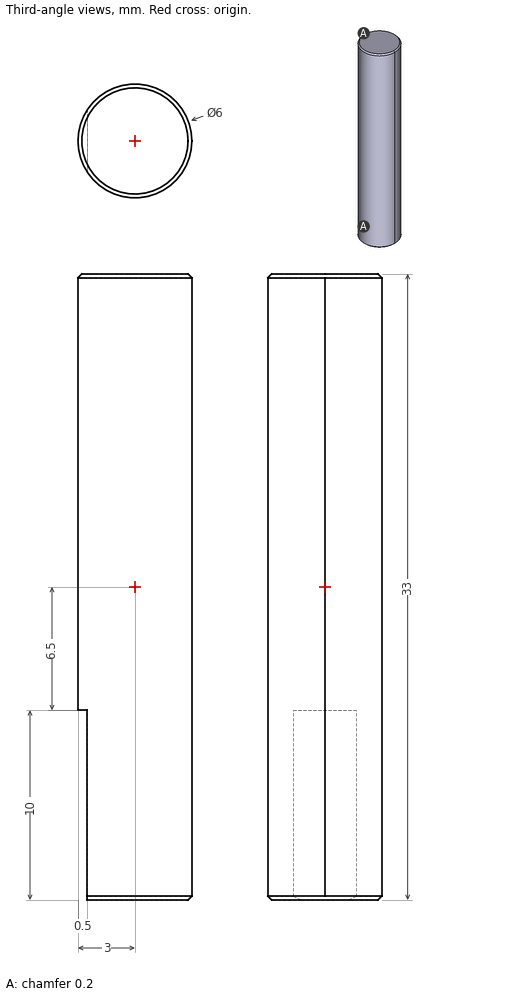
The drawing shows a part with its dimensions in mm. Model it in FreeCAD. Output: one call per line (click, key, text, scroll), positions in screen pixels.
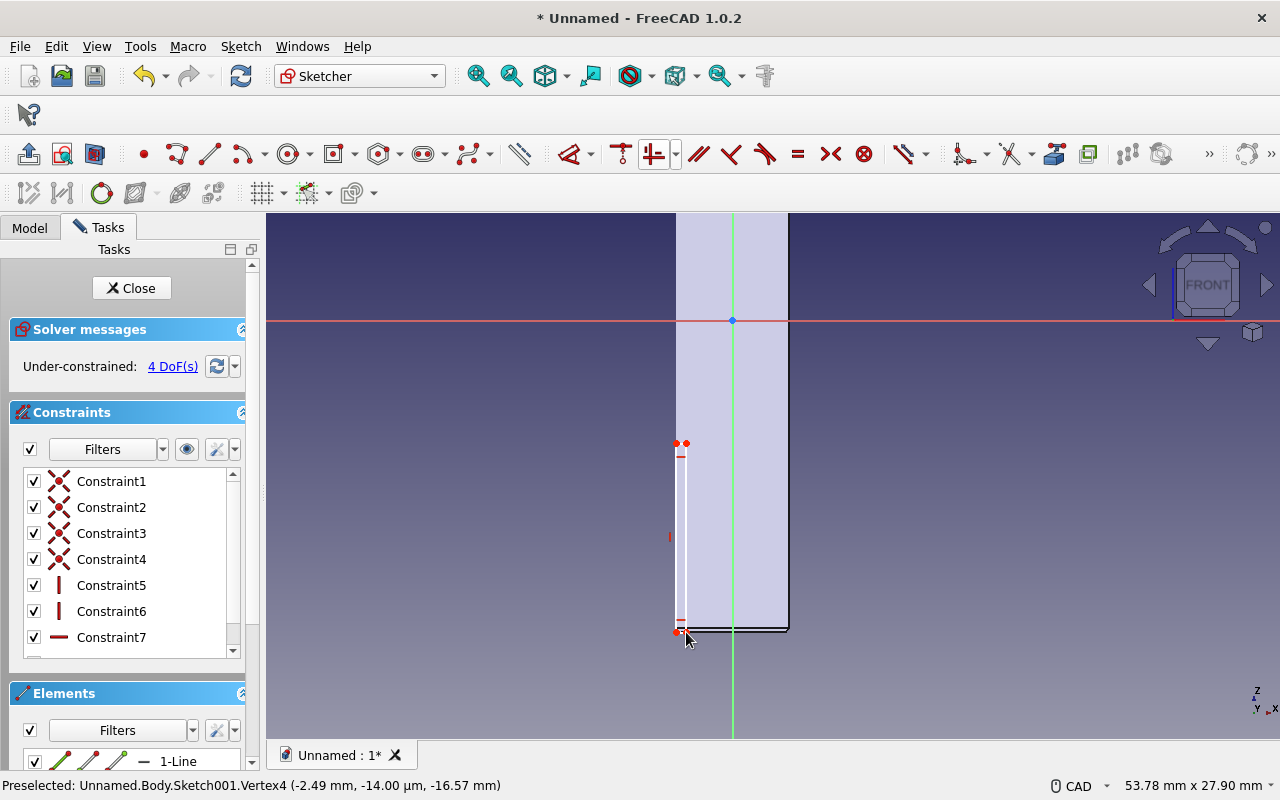
click(568, 154)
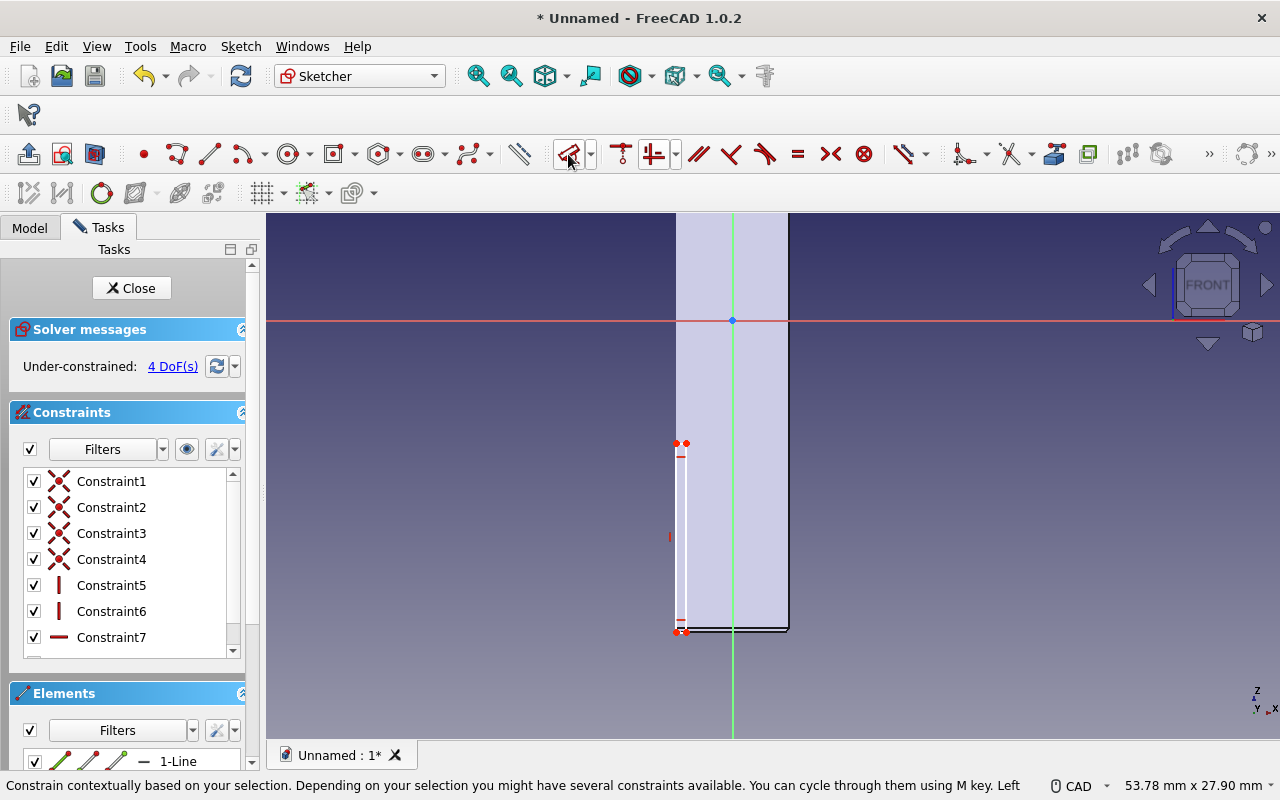
scroll(676, 500, up, 2)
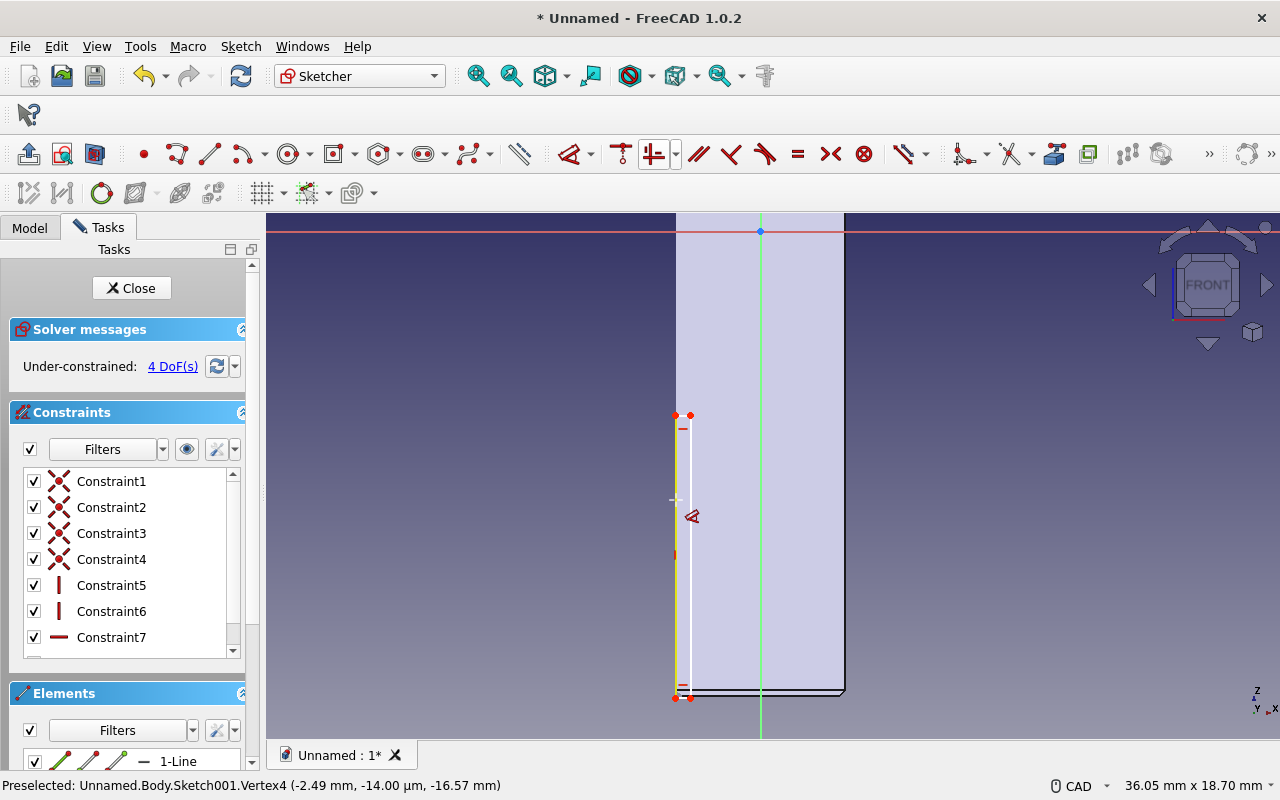
click(676, 500)
click(642, 557)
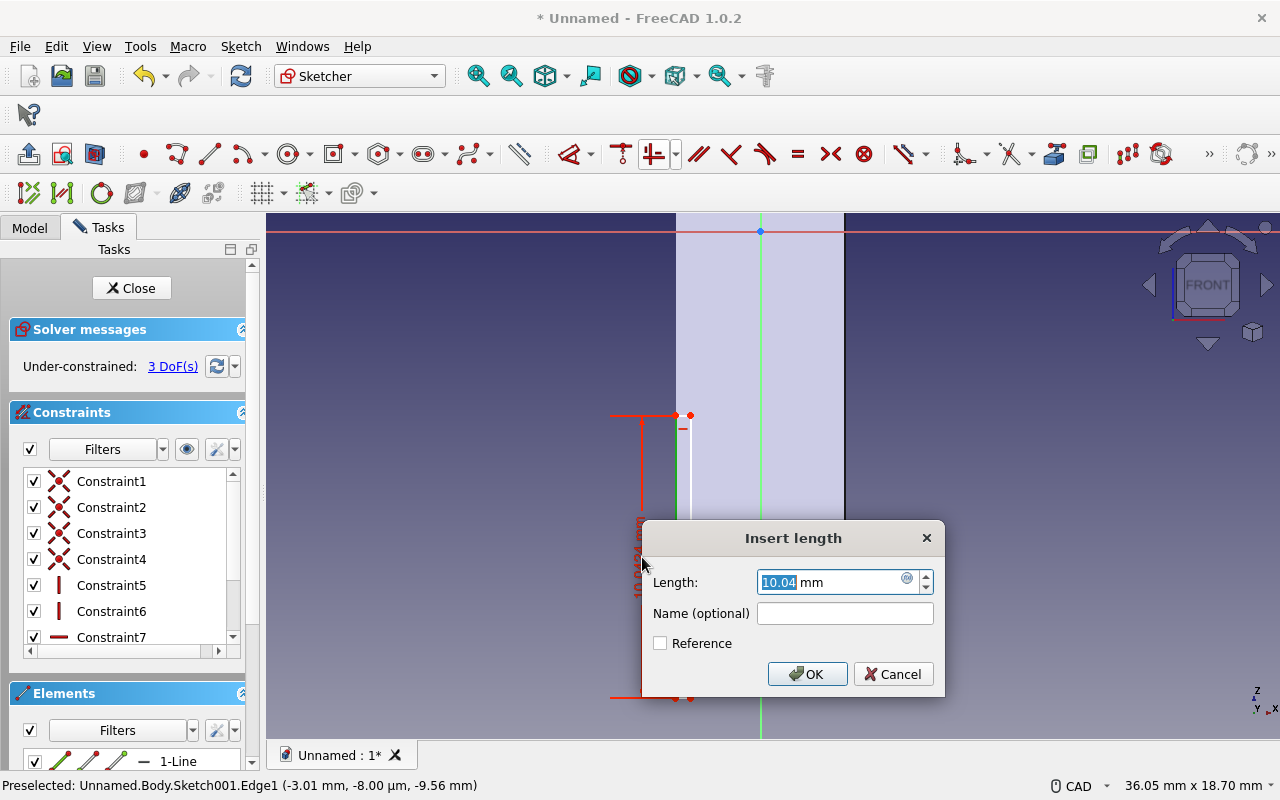
text(10)
key(Return)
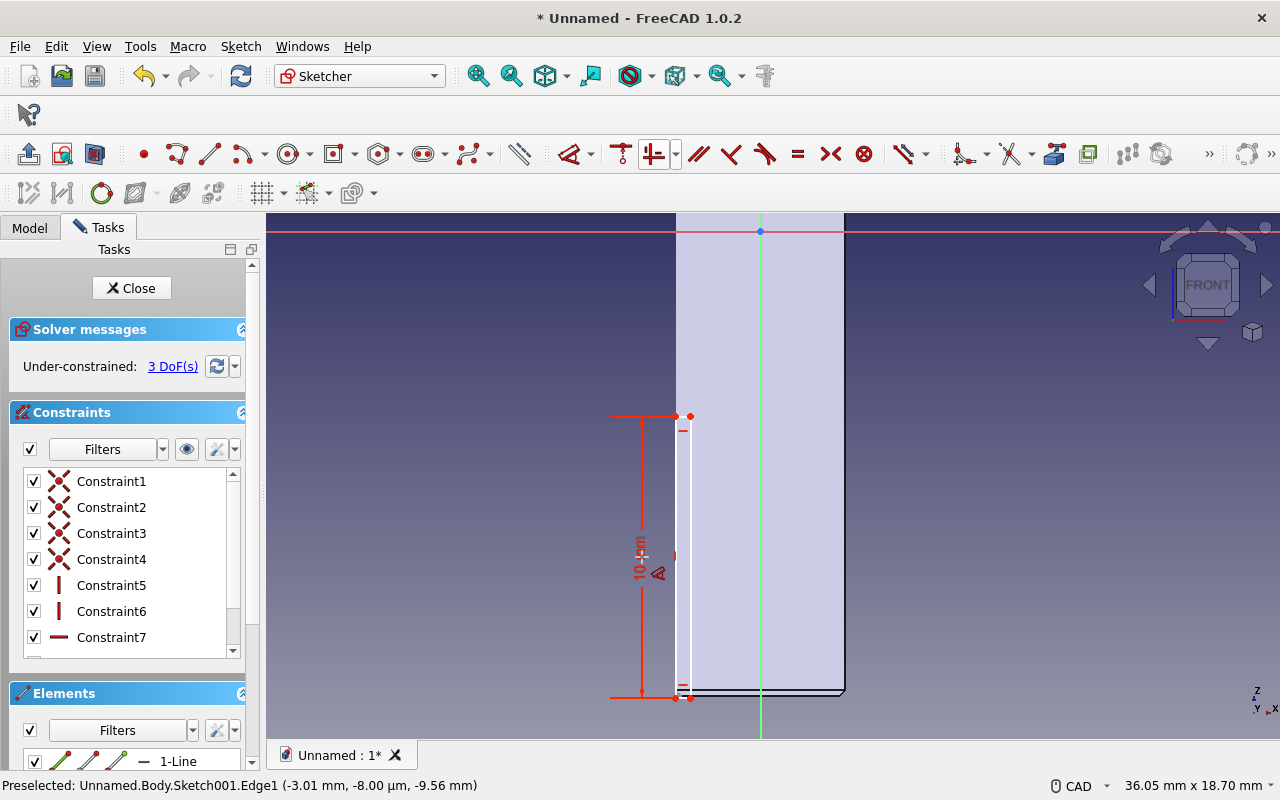
click(676, 417)
click(718, 451)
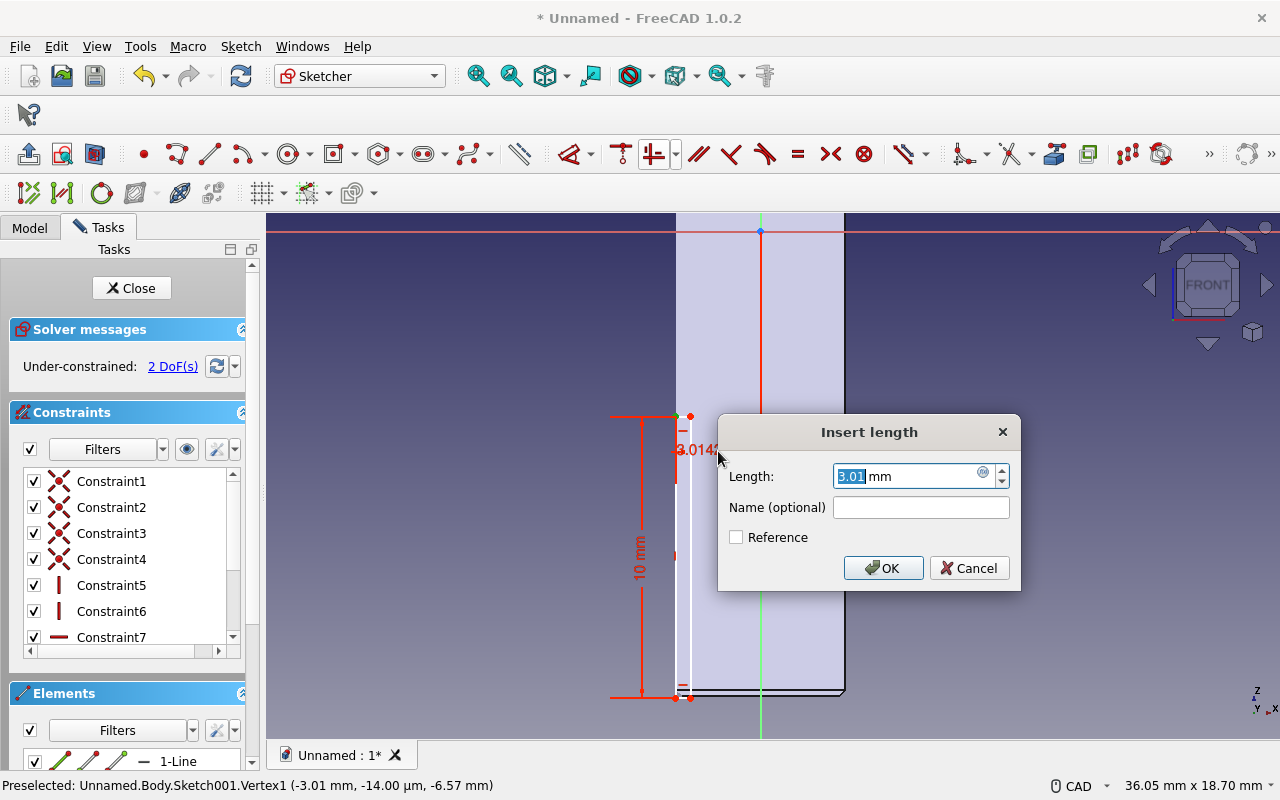
text(3)
key(Return)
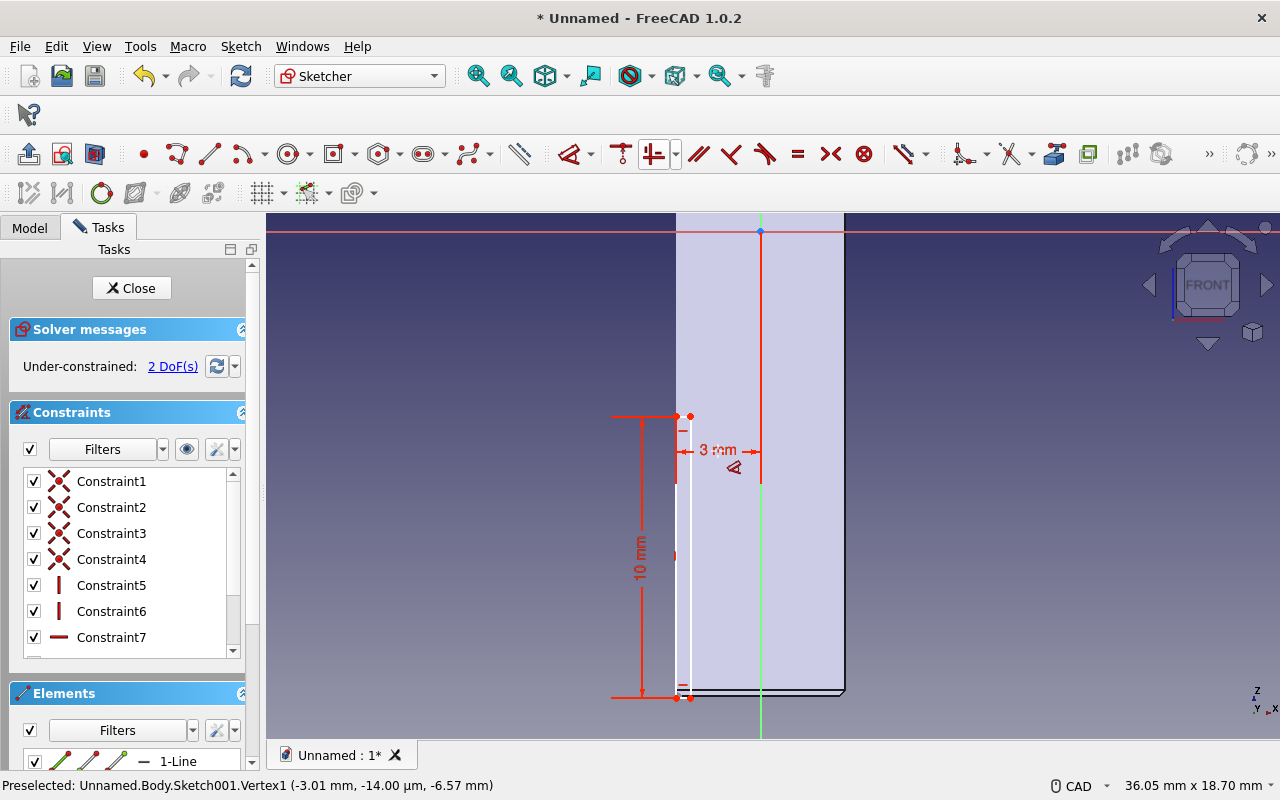
scroll(684, 698, up, 6)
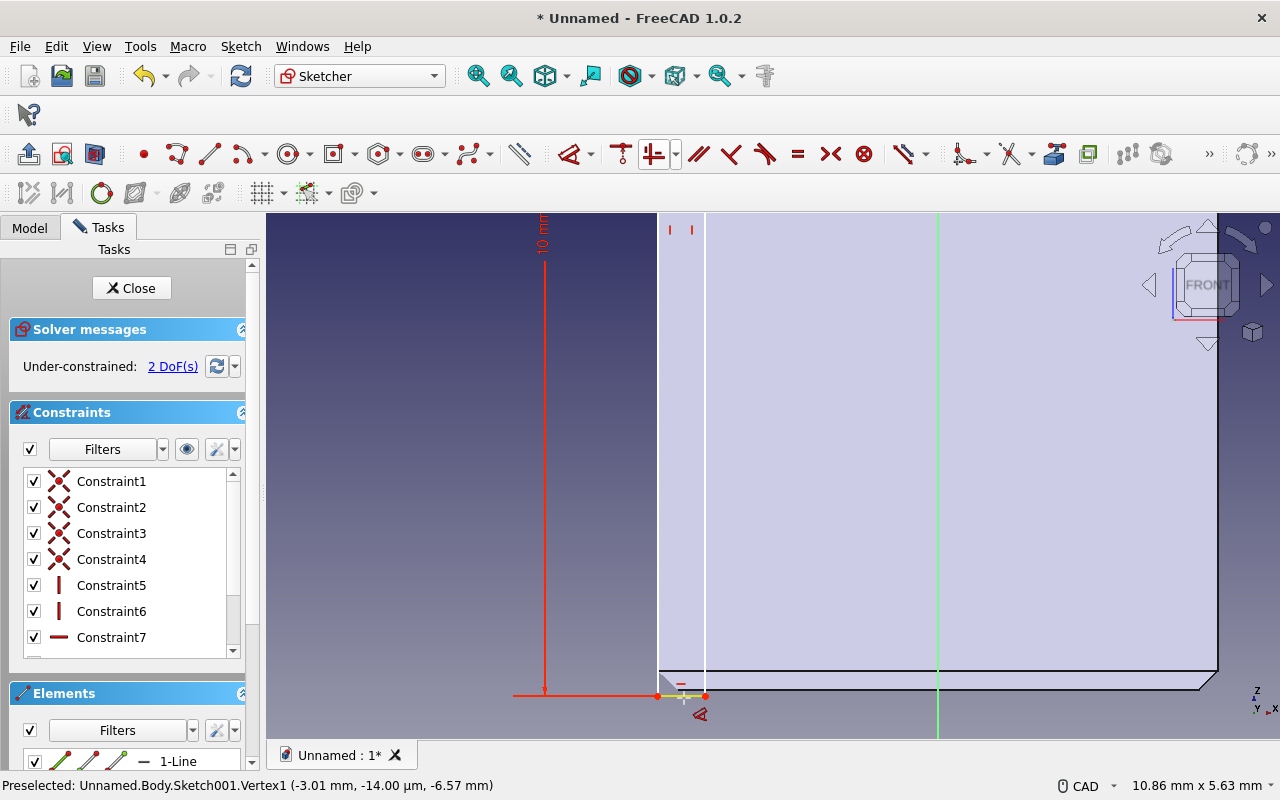
click(681, 696)
click(681, 662)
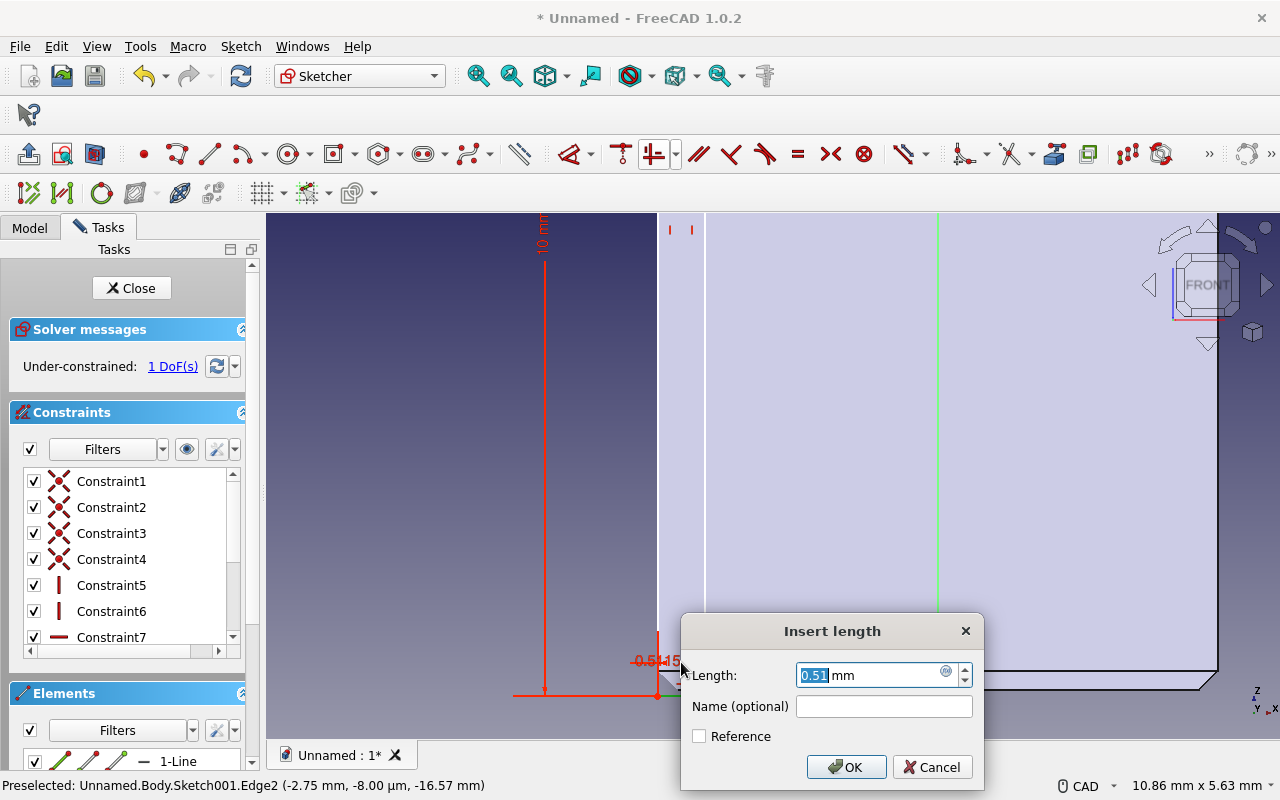
text(0.5)
key(Return)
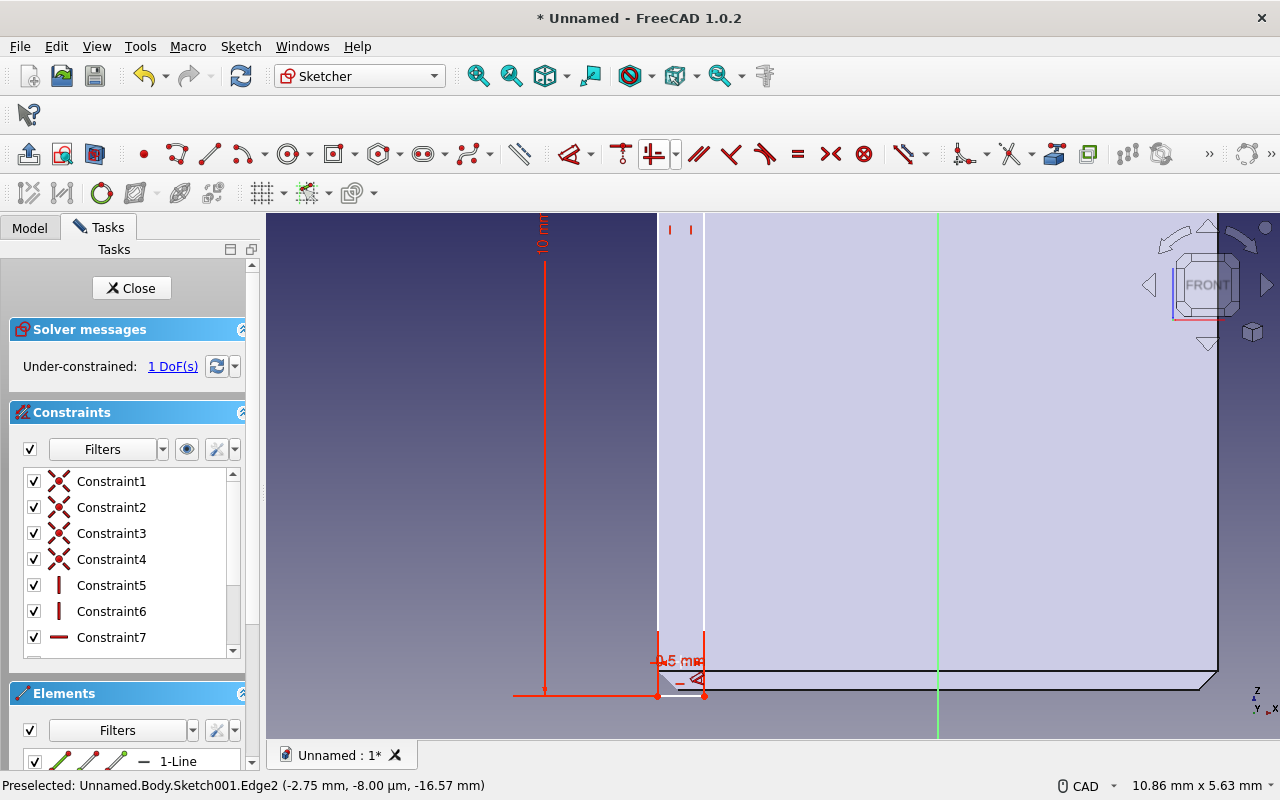
scroll(681, 617, down, 8)